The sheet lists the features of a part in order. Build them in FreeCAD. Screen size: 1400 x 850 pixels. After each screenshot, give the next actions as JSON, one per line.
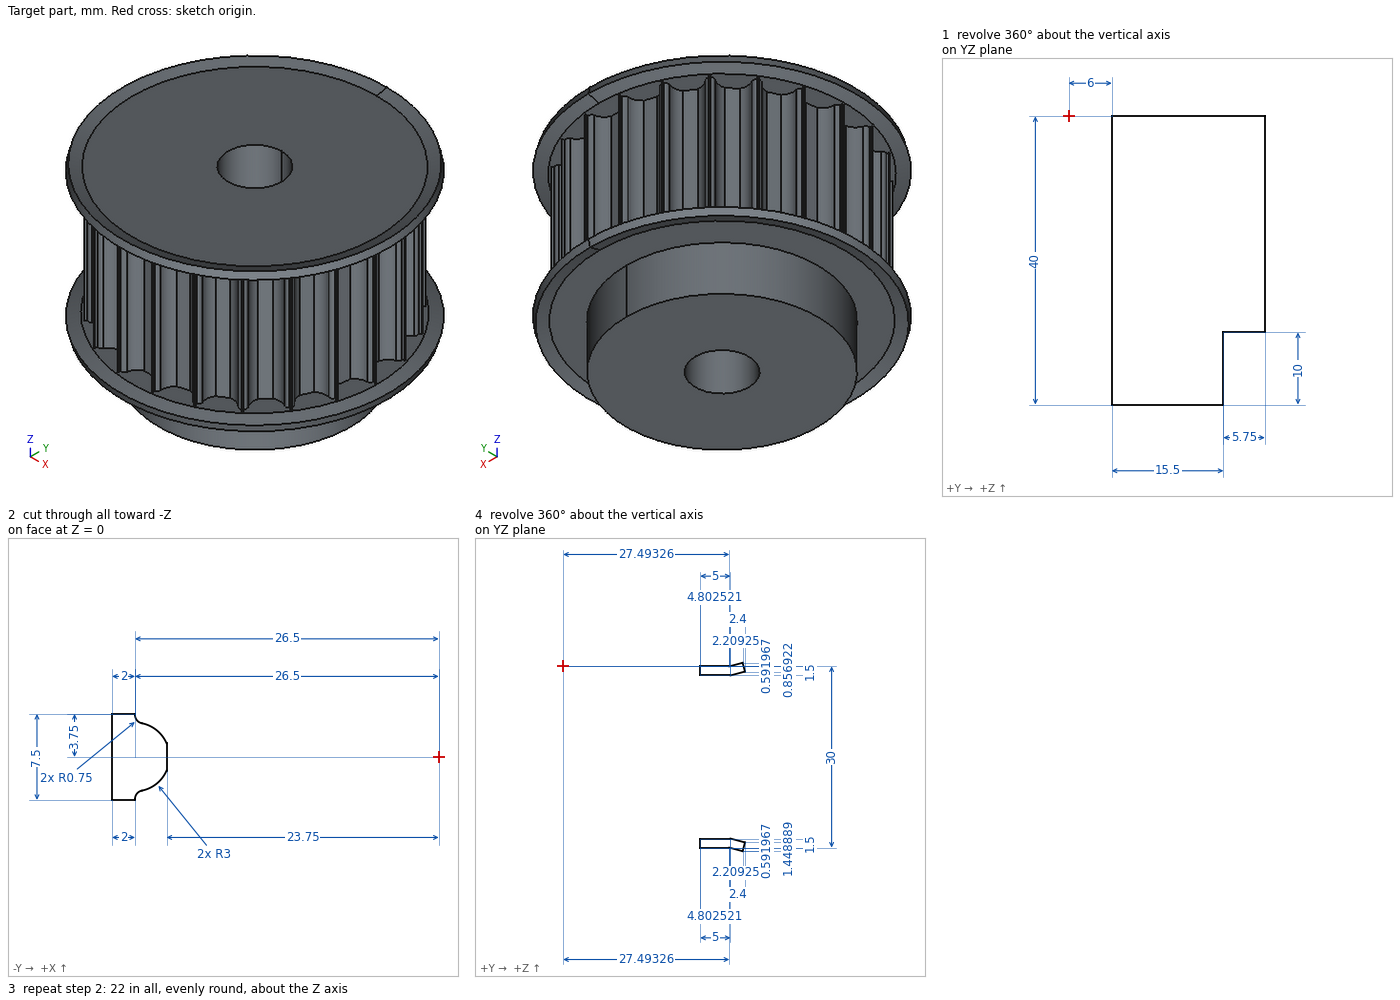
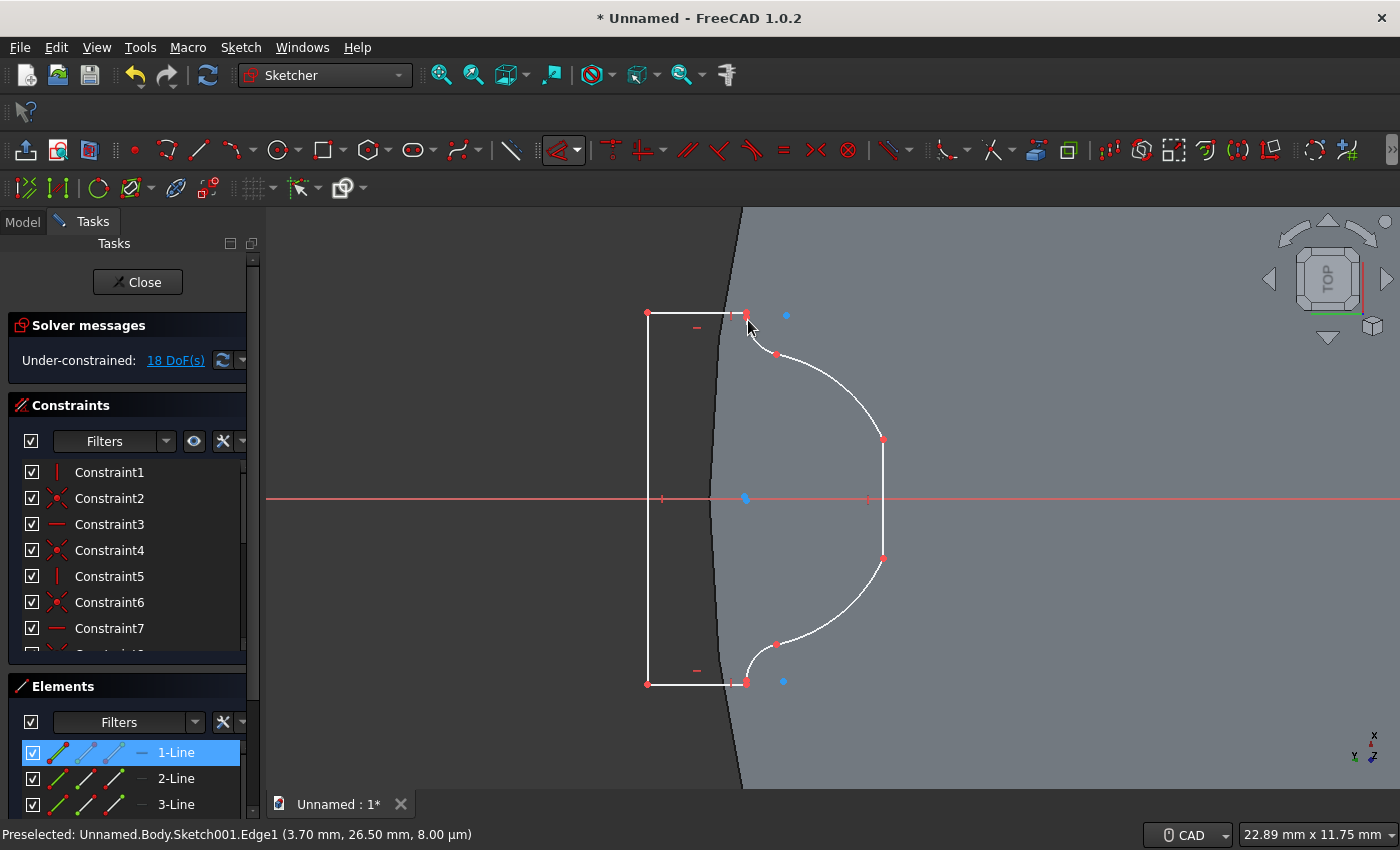
{"action": "left_click", "coordinate": [750, 332]}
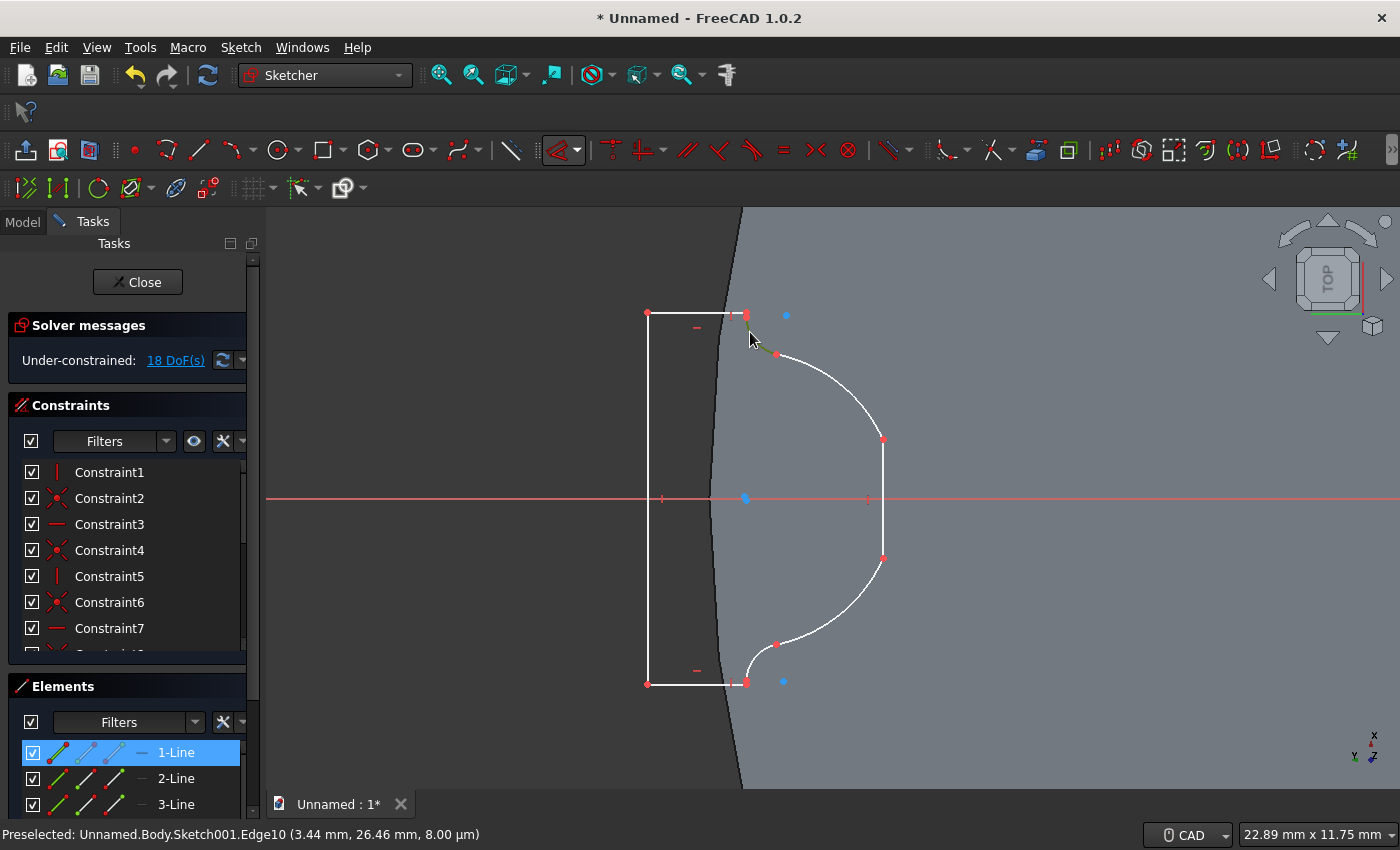
{"action": "left_click", "coordinate": [752, 150]}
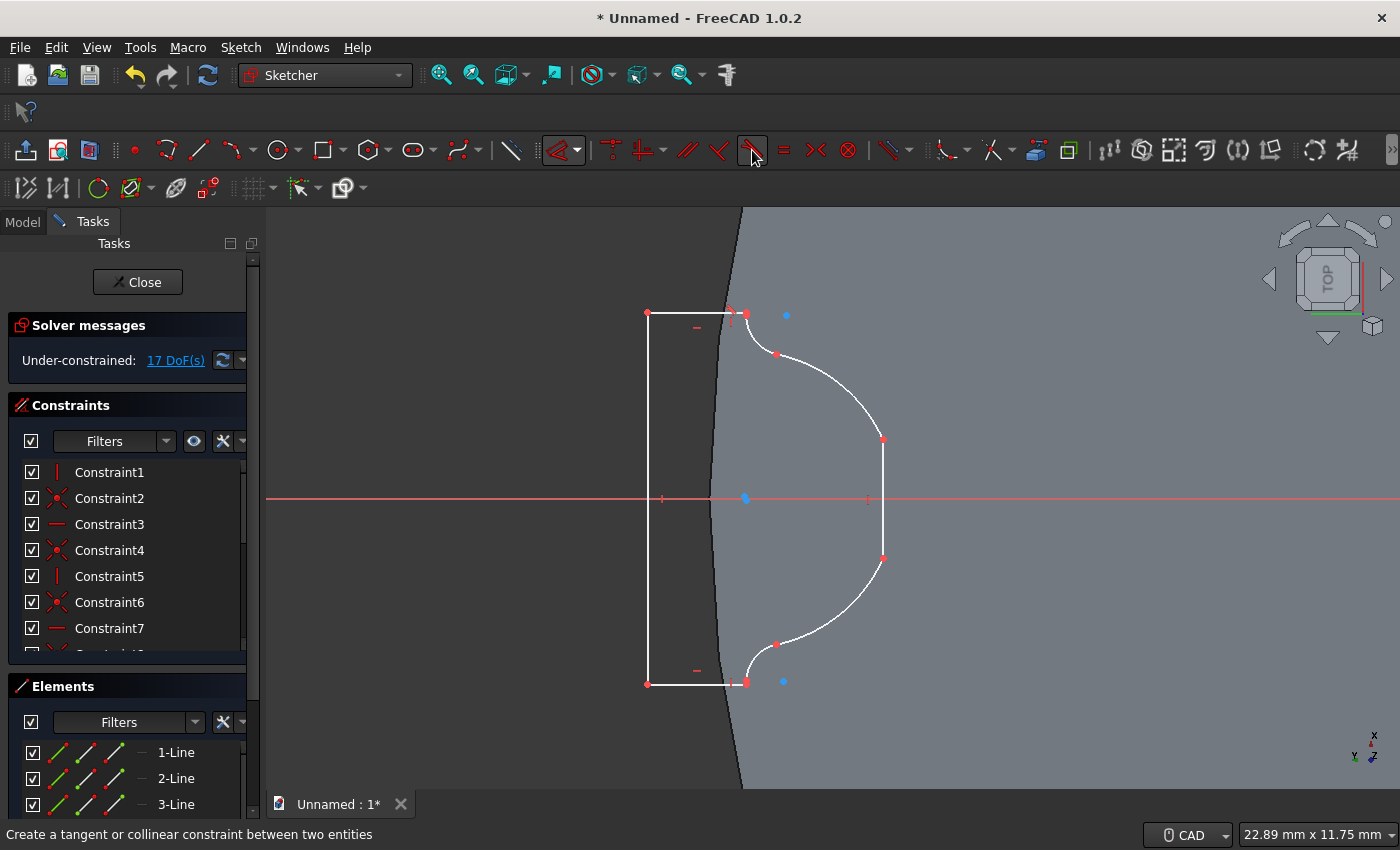
{"action": "scroll", "coordinate": [747, 683], "scroll_direction": "up", "scroll_amount": 10}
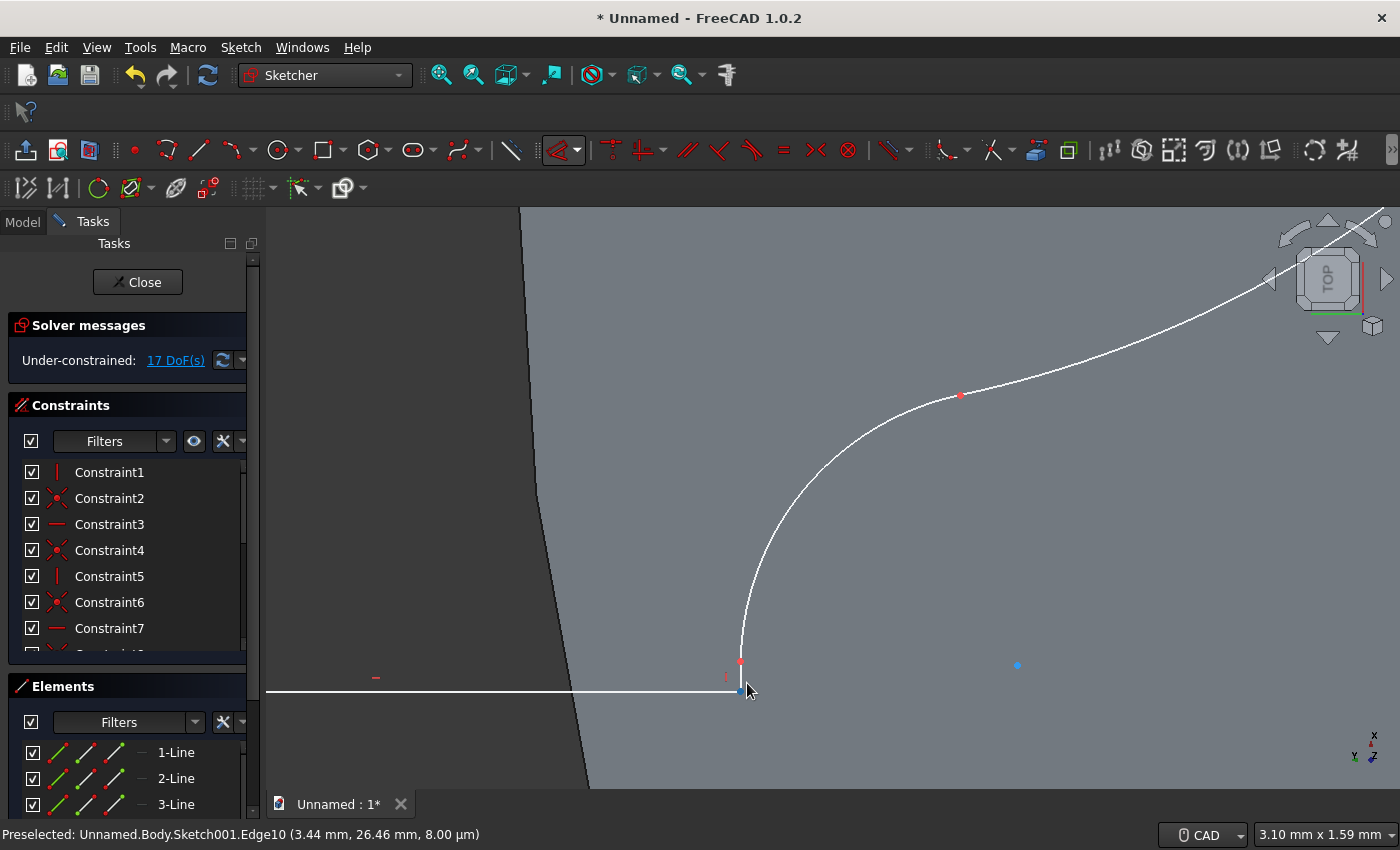
{"action": "left_click", "coordinate": [741, 676]}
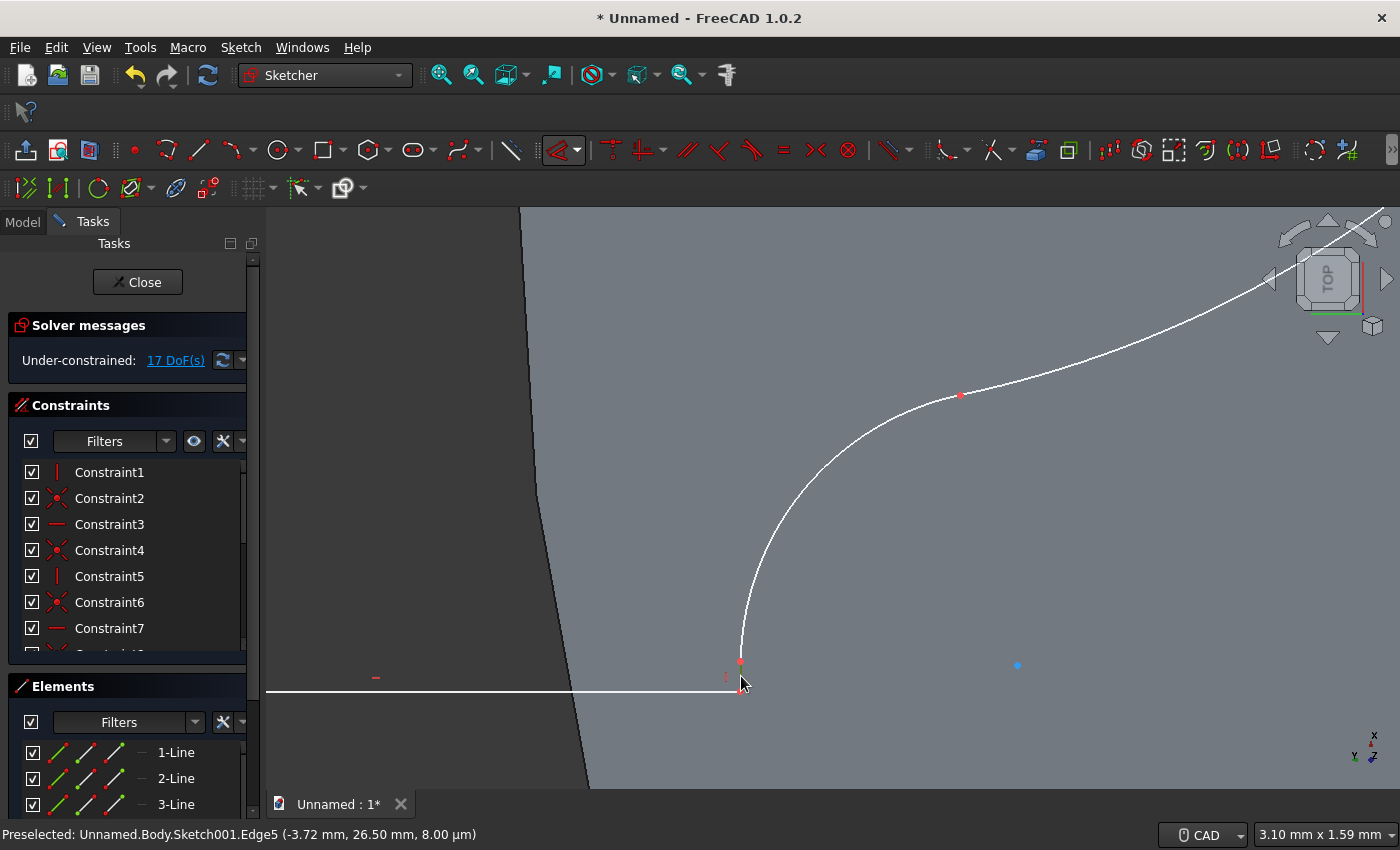
{"action": "scroll", "coordinate": [747, 683], "scroll_direction": "down", "scroll_amount": 10}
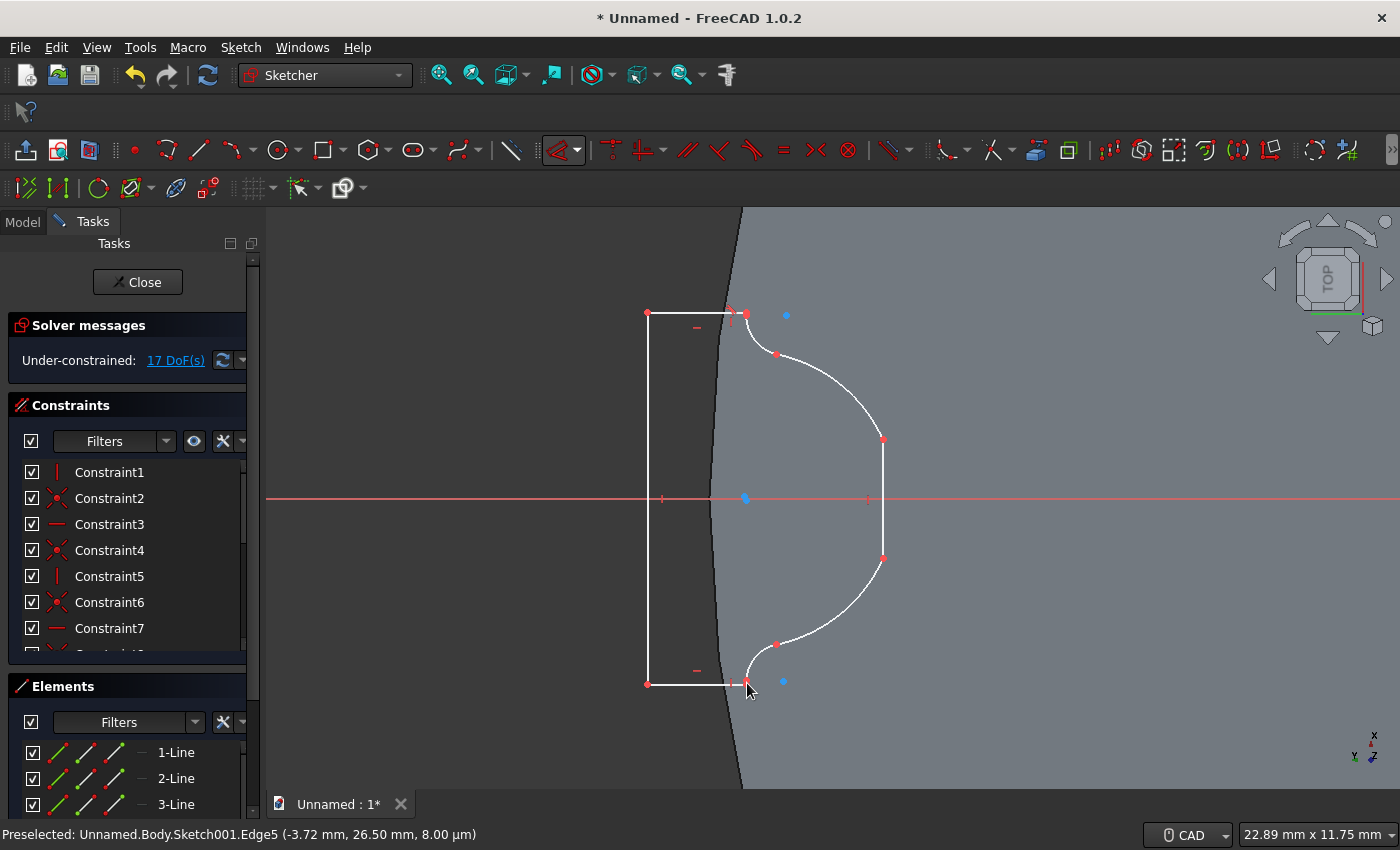
{"action": "left_click", "coordinate": [762, 651]}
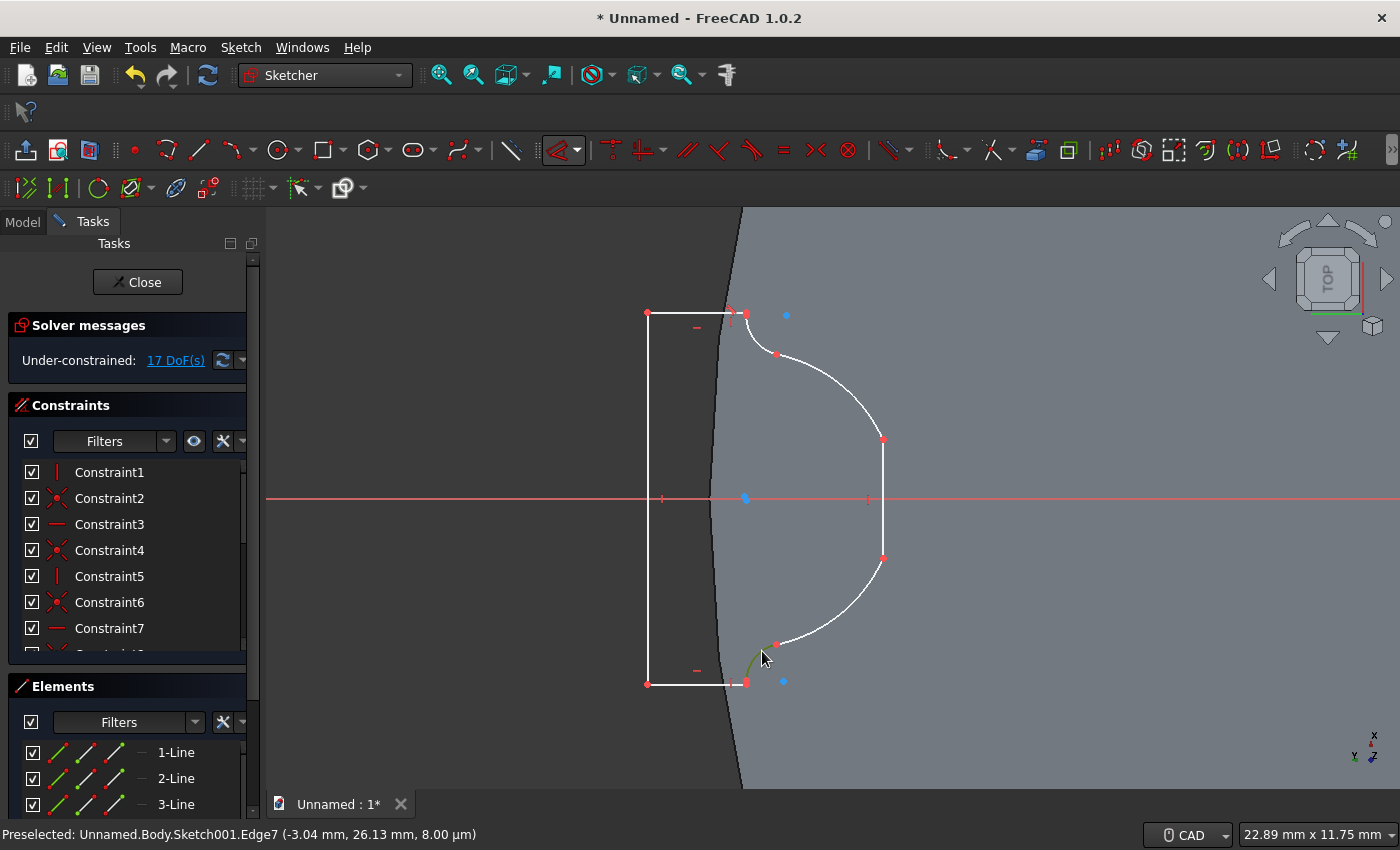
{"action": "left_click", "coordinate": [752, 150]}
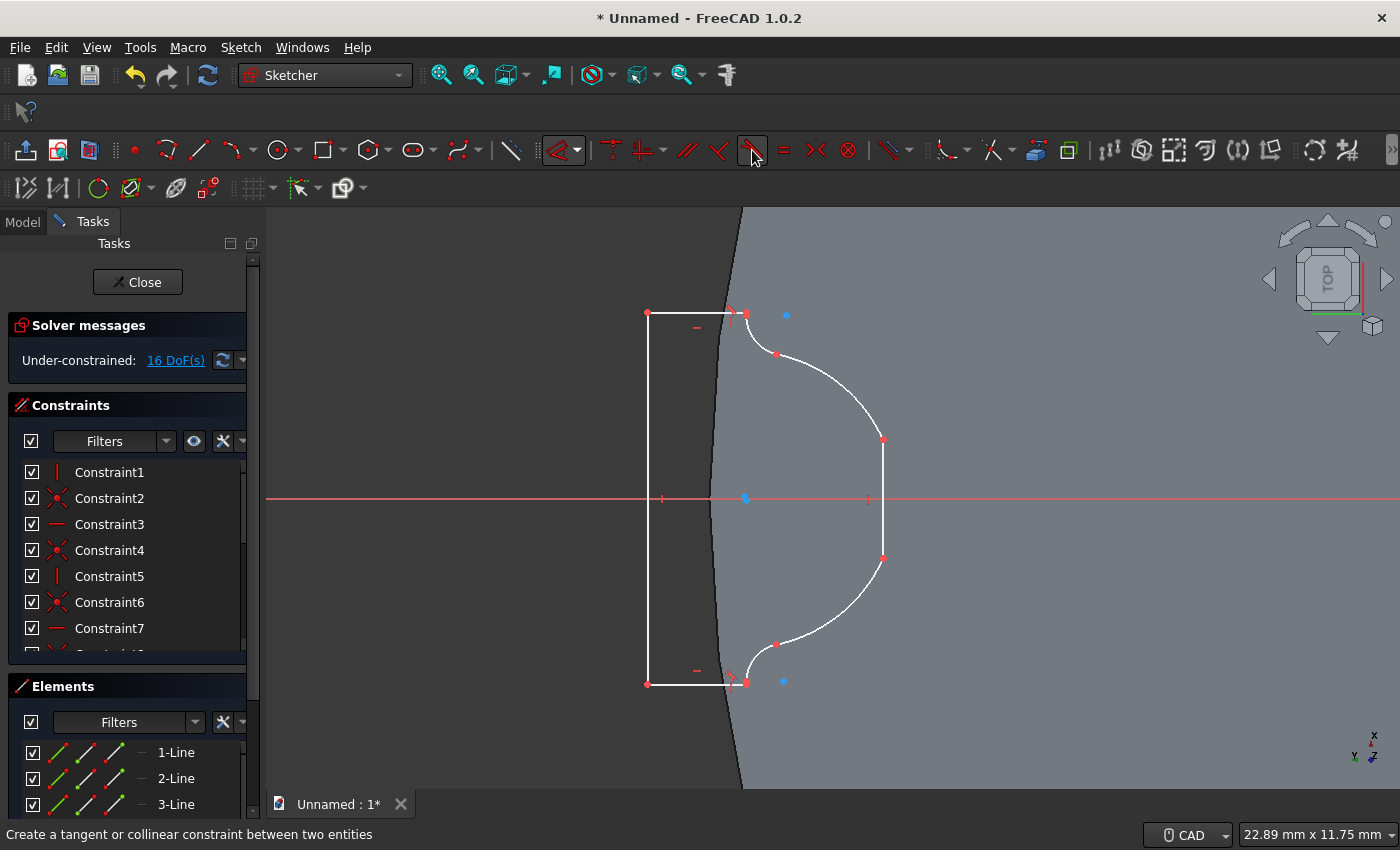
{"action": "left_click", "coordinate": [762, 651]}